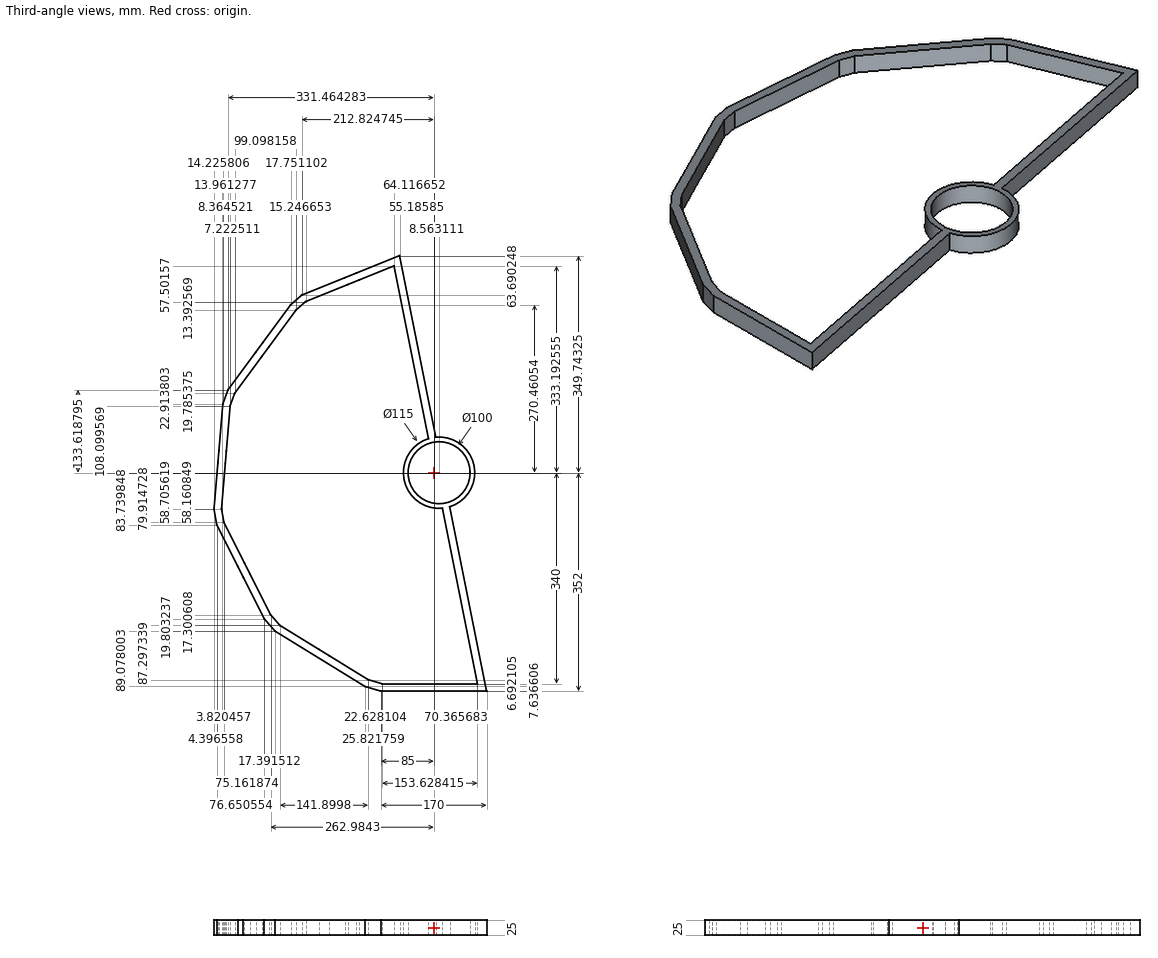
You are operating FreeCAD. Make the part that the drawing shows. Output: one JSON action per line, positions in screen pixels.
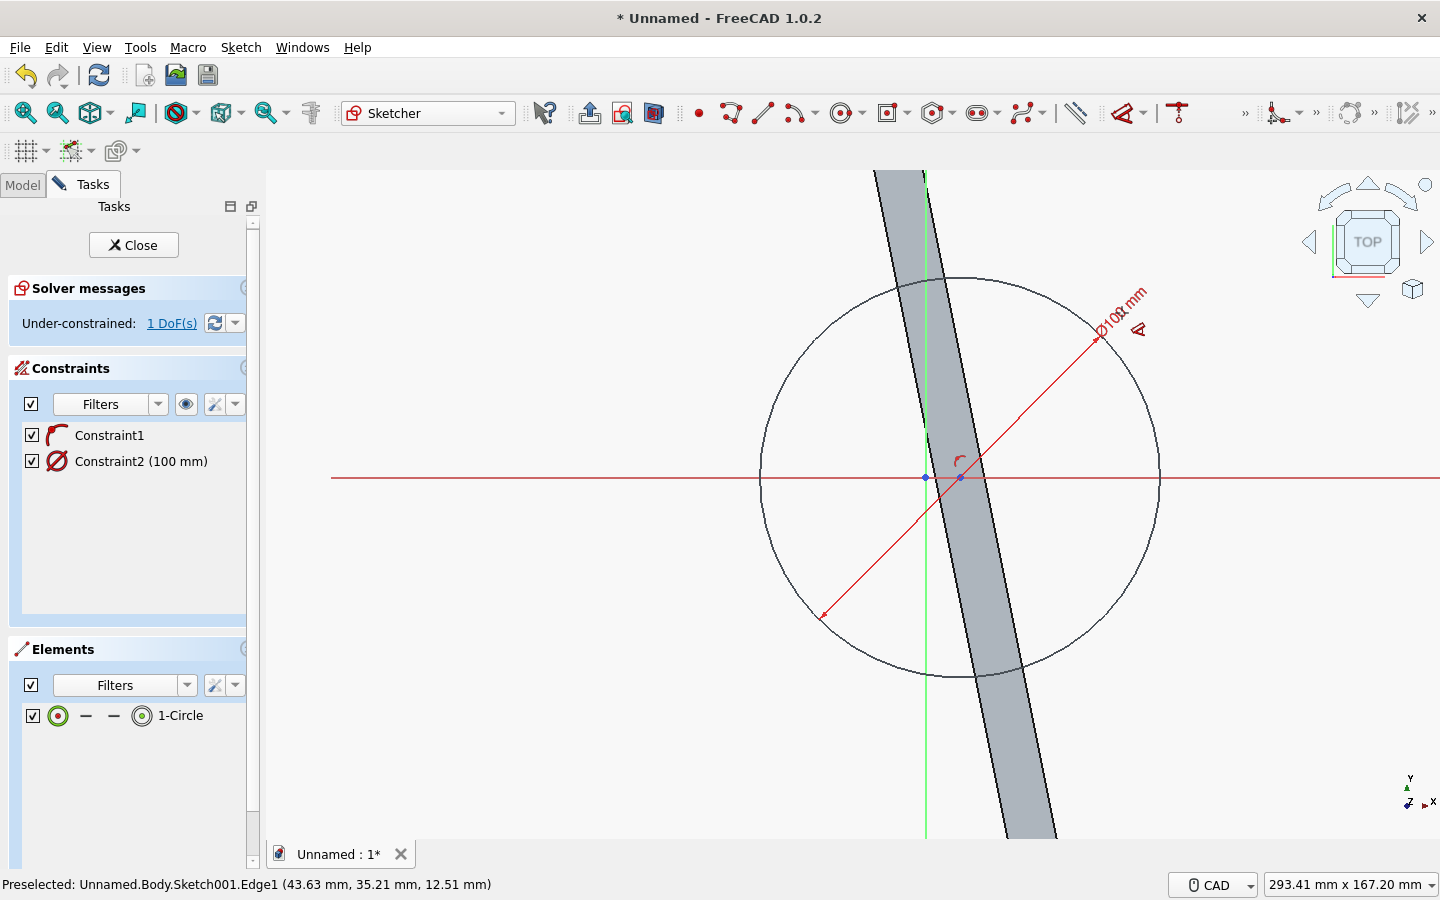
{"action": "left_click", "coordinate": [960, 478]}
{"action": "left_click", "coordinate": [943, 512]}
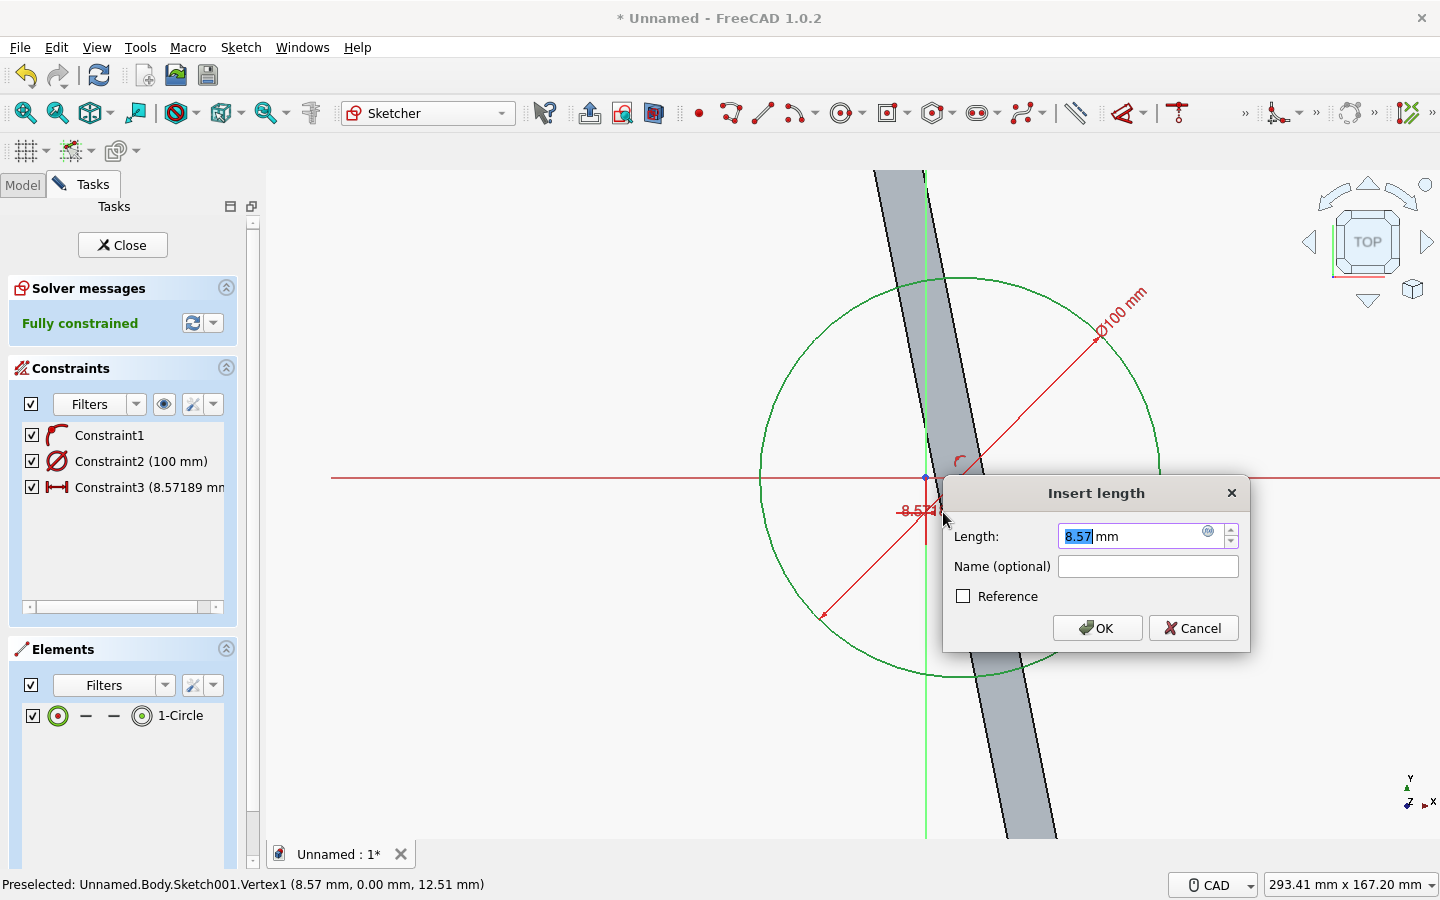
{"action": "type", "text": "8.563111"}
{"action": "key", "text": "Return"}
{"action": "key", "text": "Escape"}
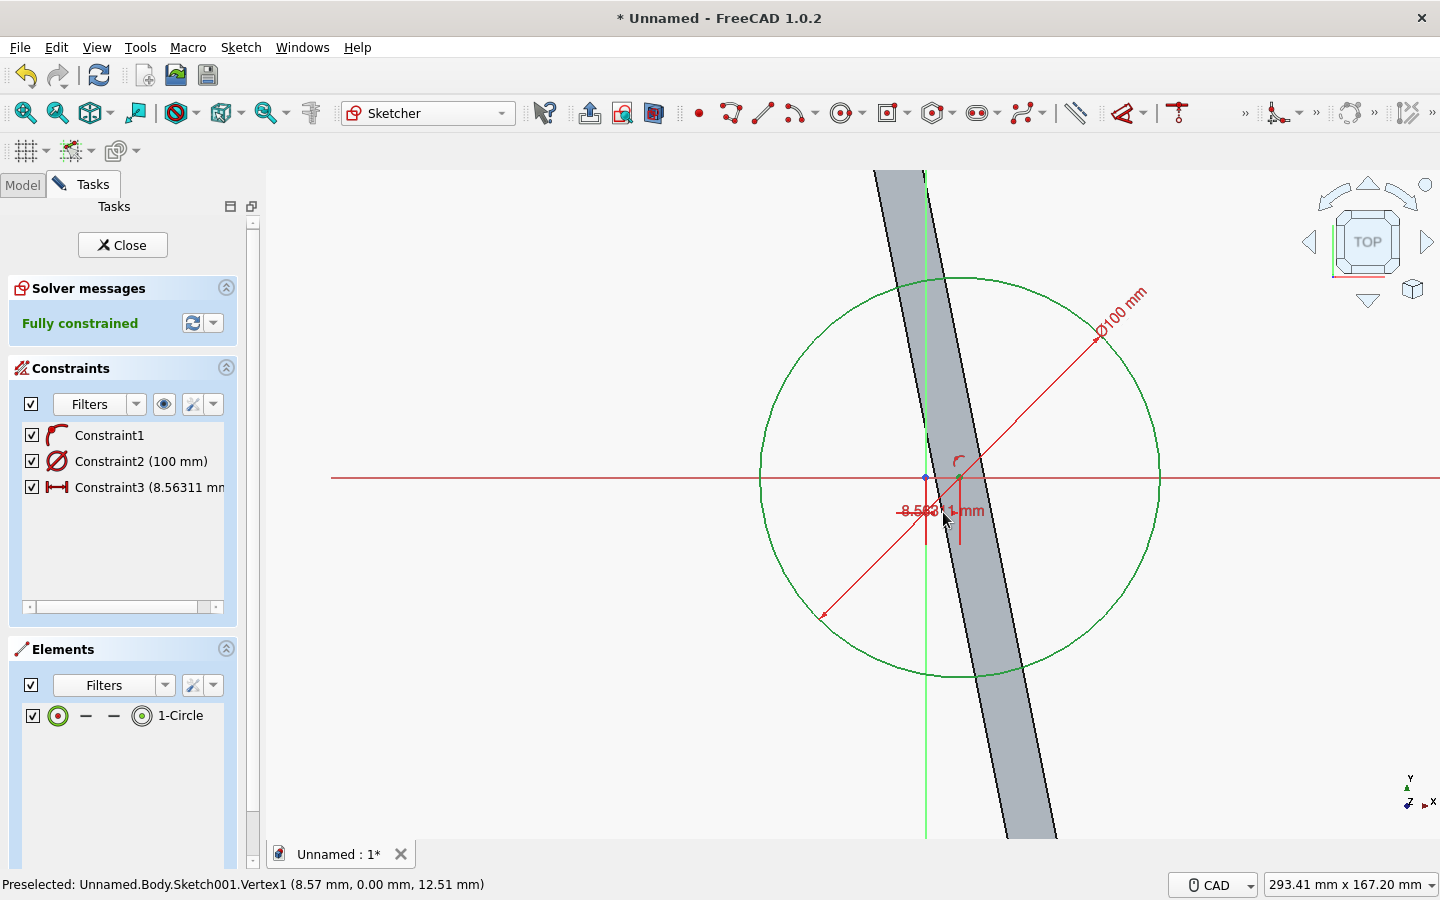
{"action": "left_click", "coordinate": [123, 245]}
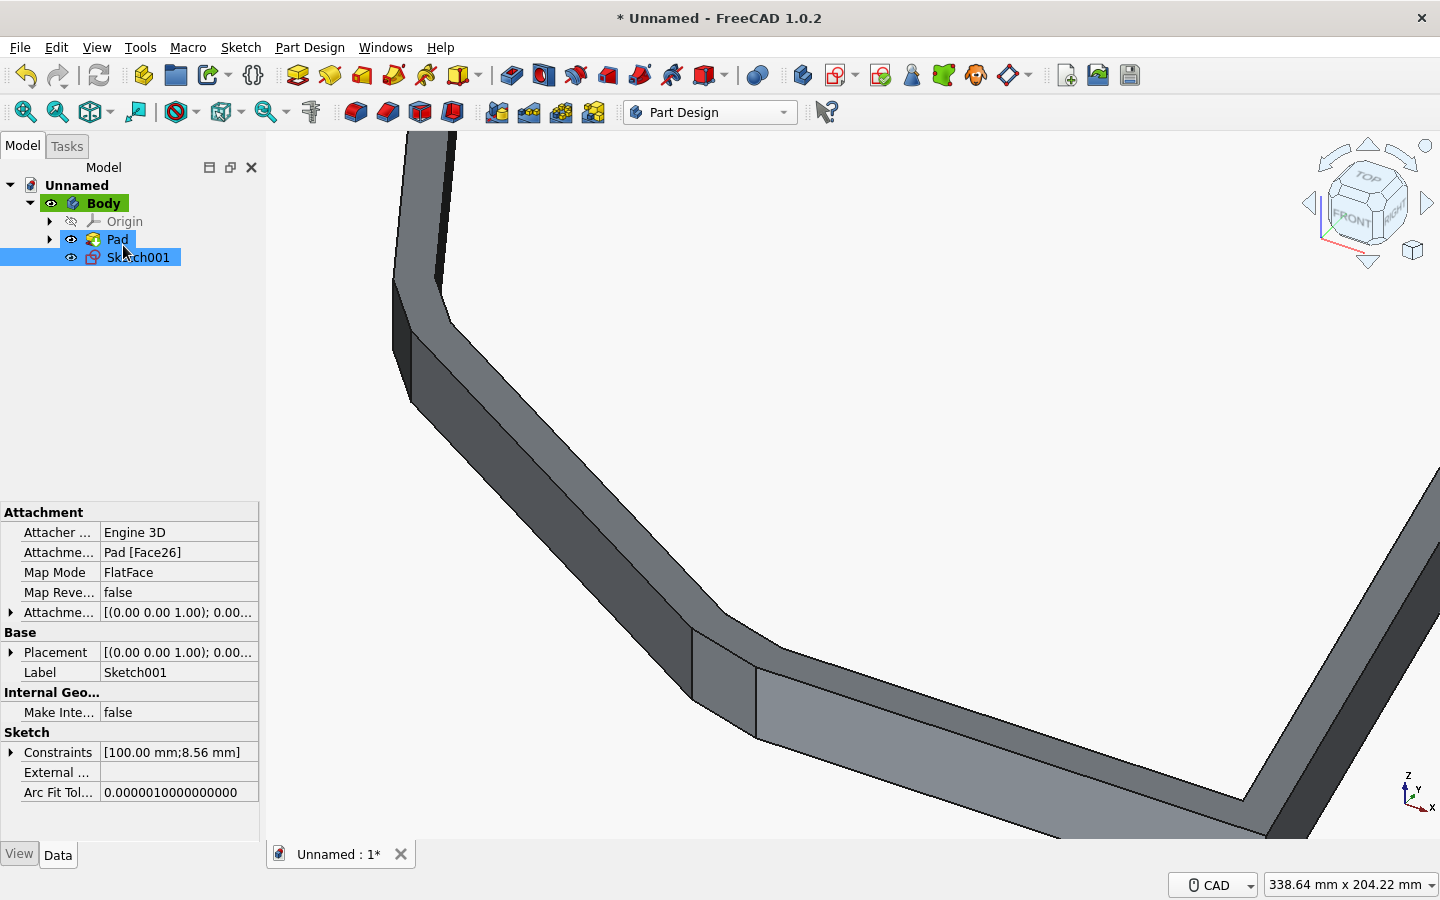
{"action": "left_click", "coordinate": [512, 76]}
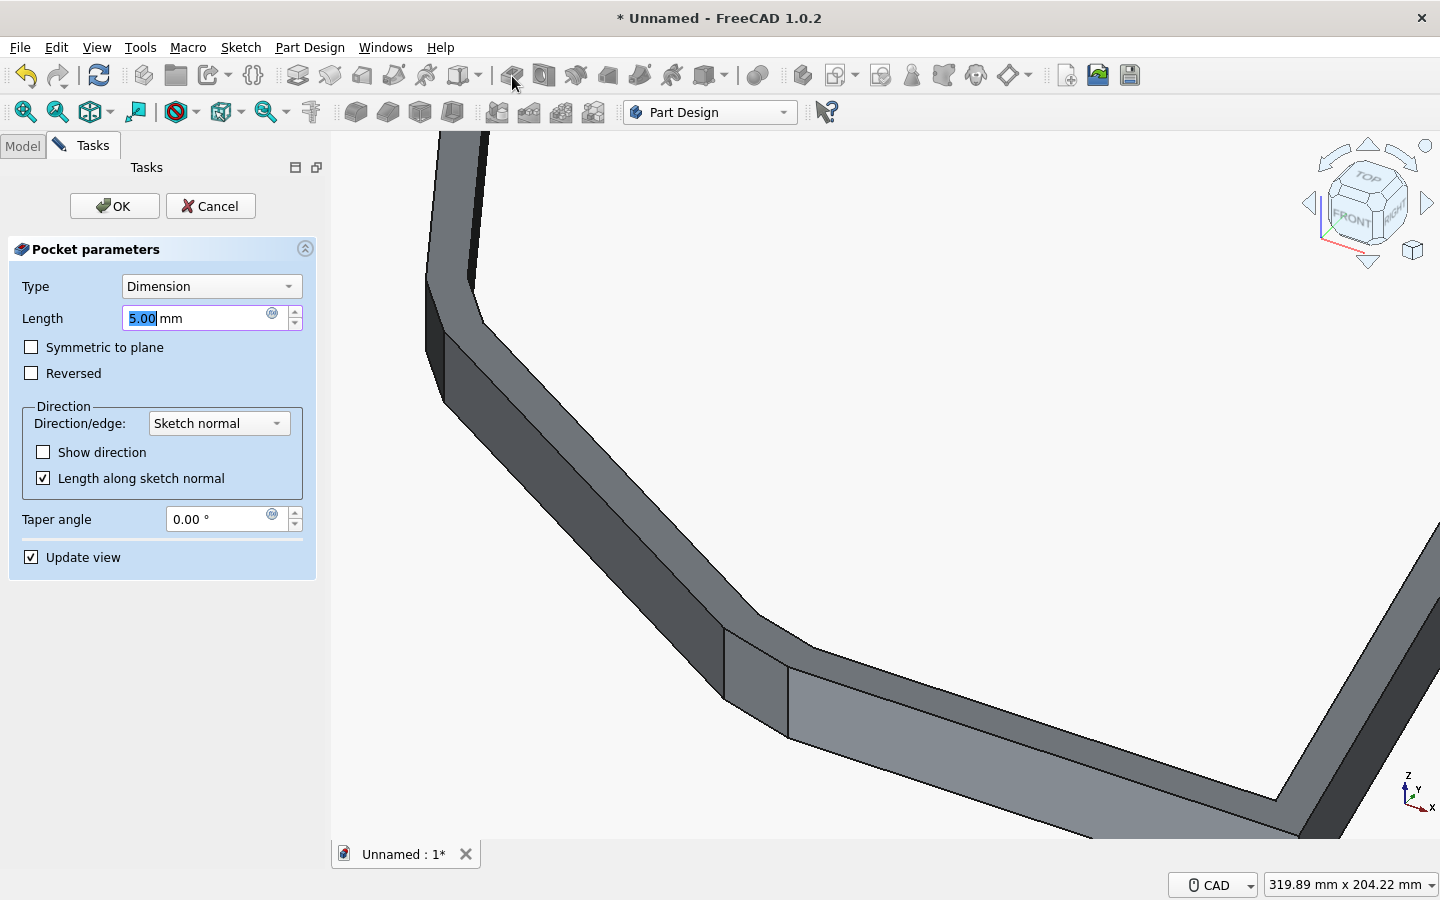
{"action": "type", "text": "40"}
{"action": "key", "text": "Tab"}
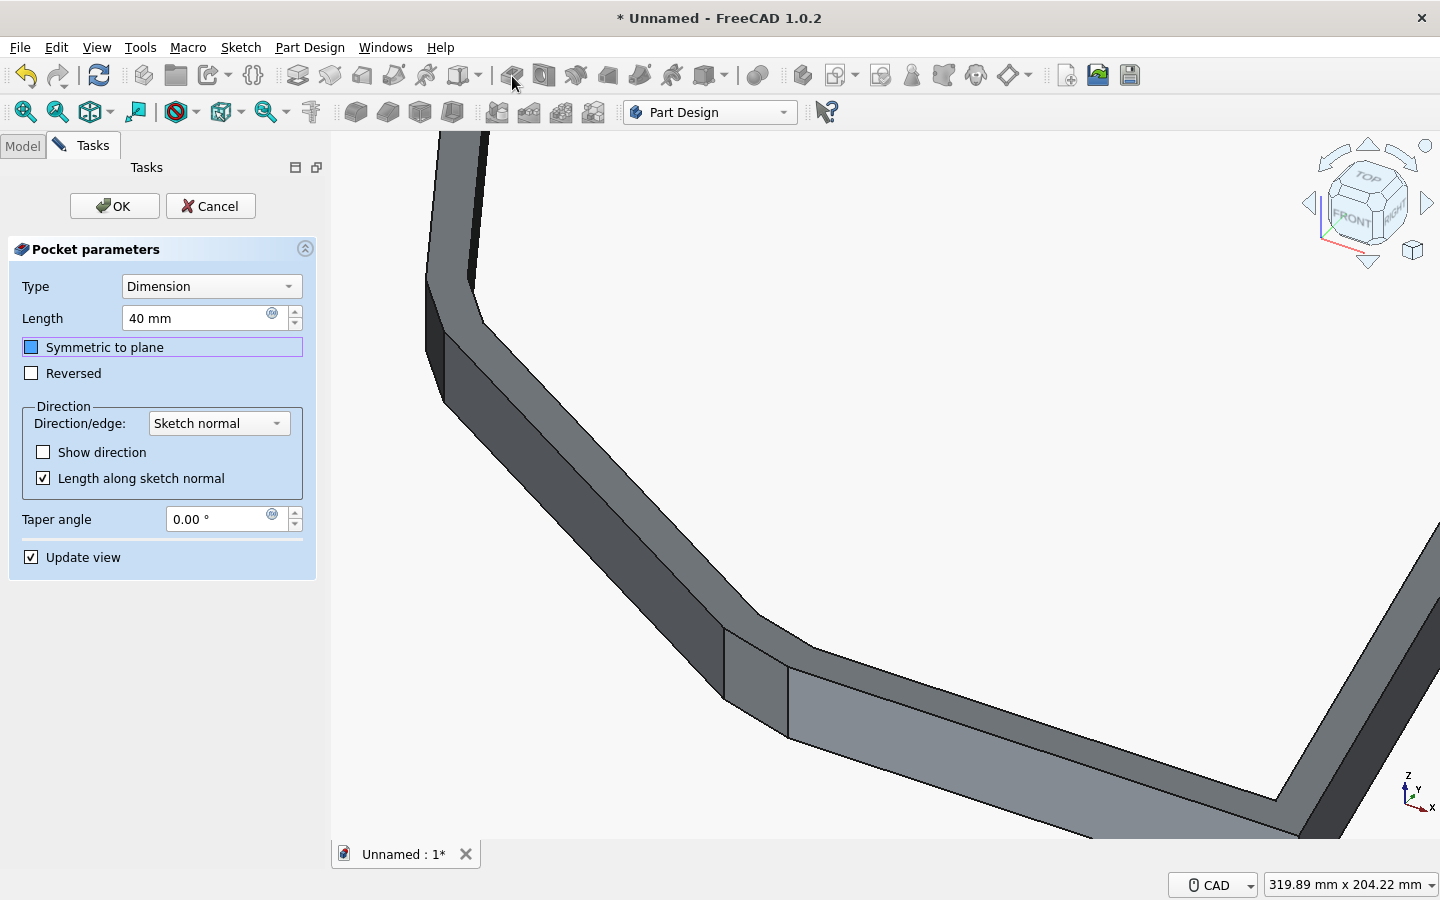
{"action": "left_click", "coordinate": [115, 206]}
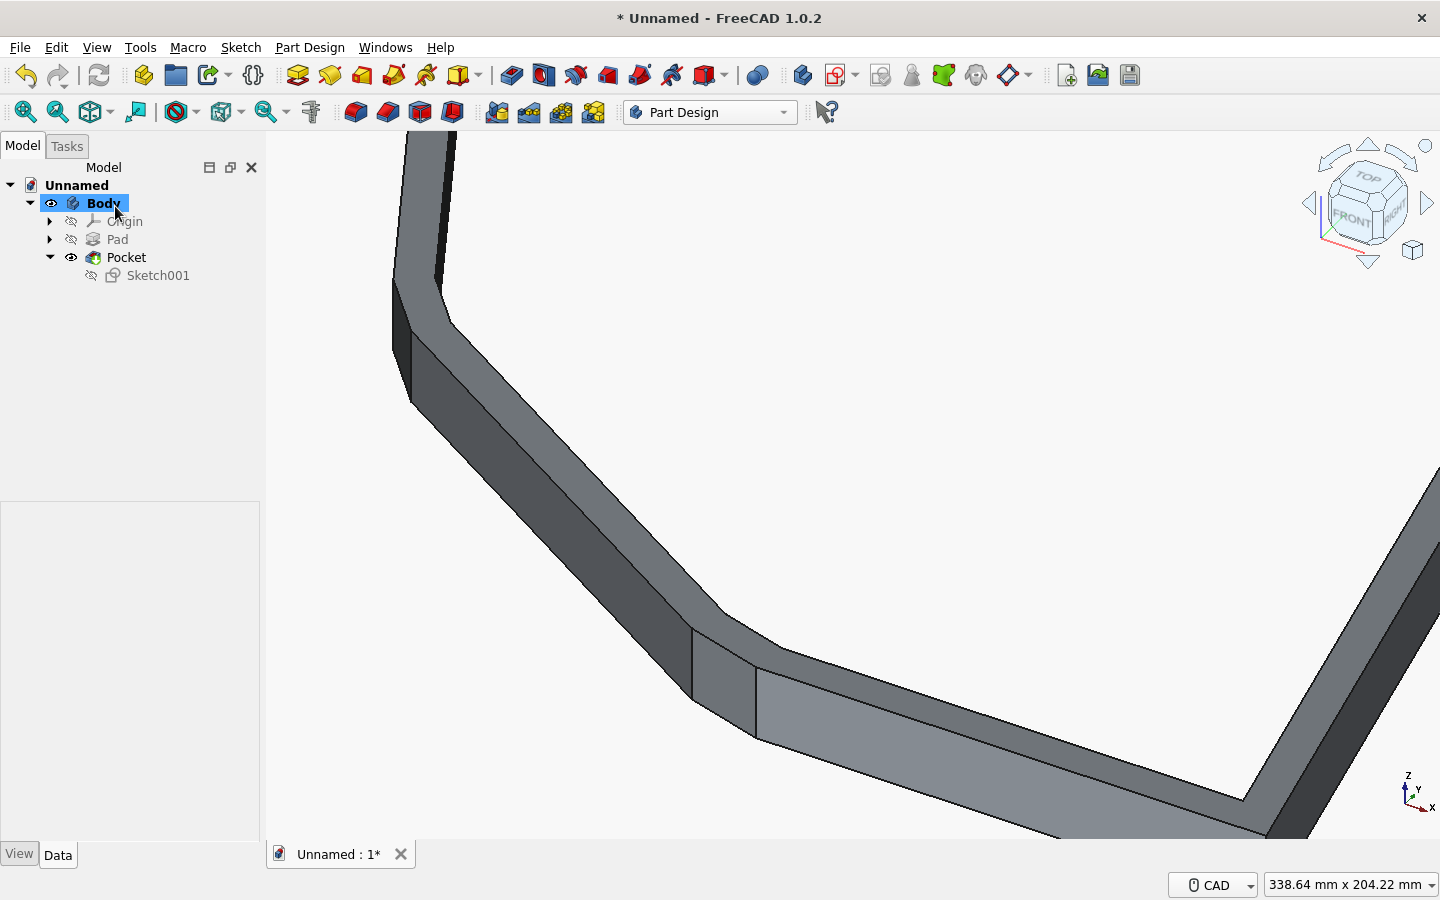
{"action": "left_click", "coordinate": [26, 112]}